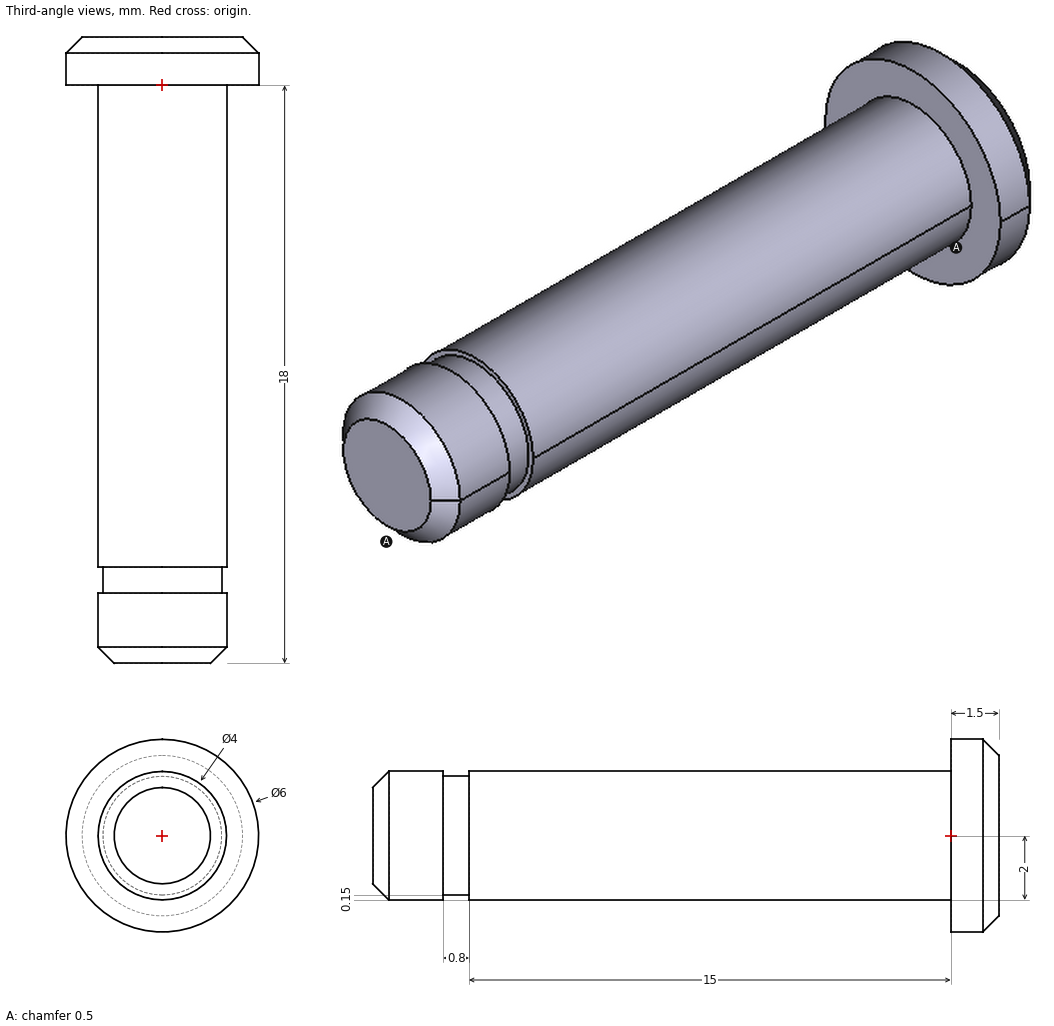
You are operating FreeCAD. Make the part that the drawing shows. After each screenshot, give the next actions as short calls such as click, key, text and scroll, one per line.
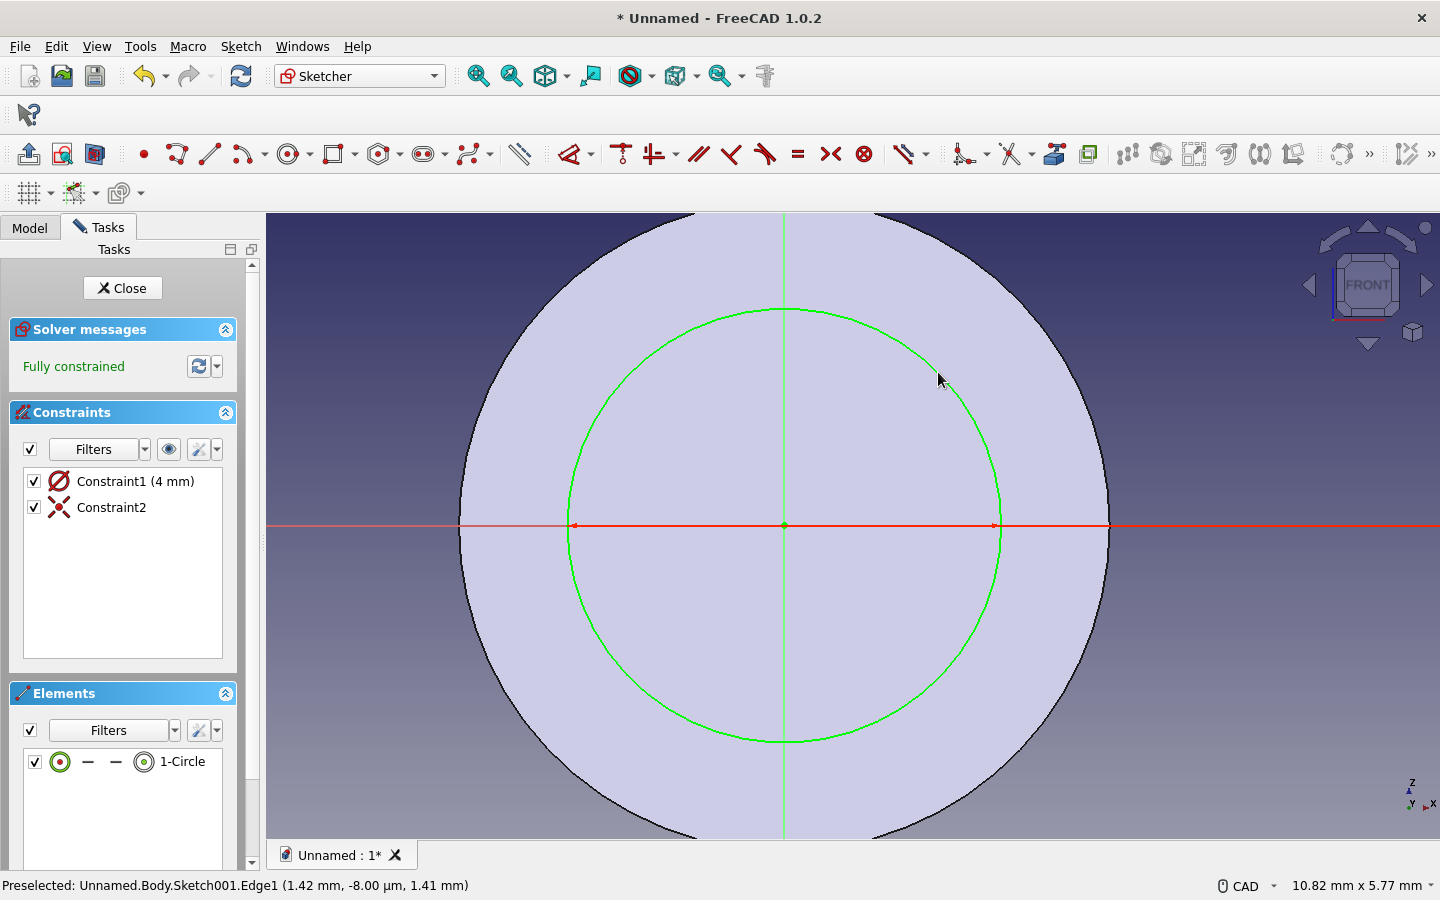
click(123, 288)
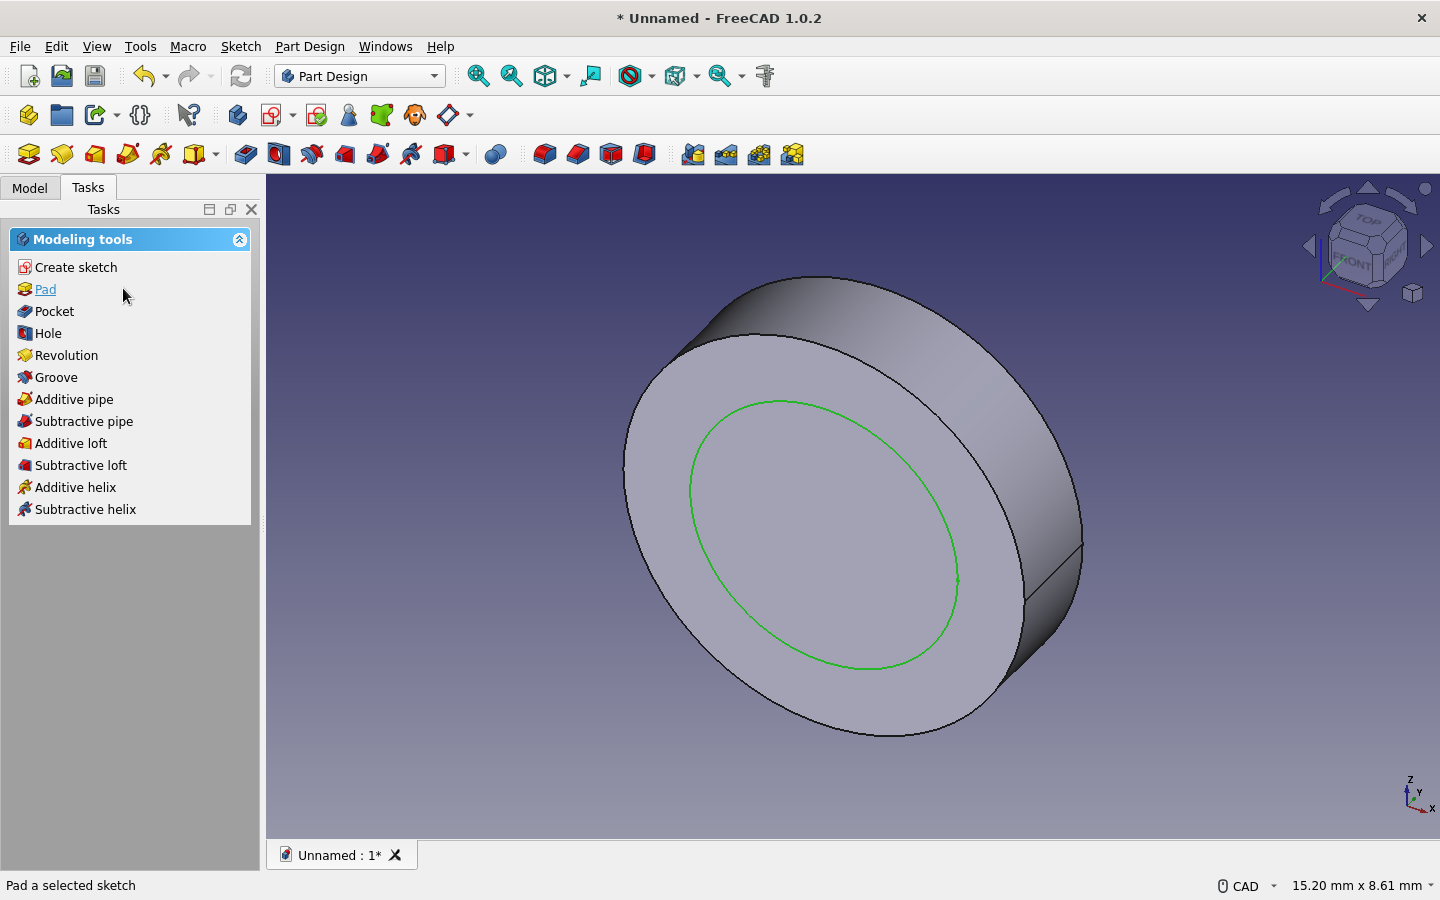
click(29, 154)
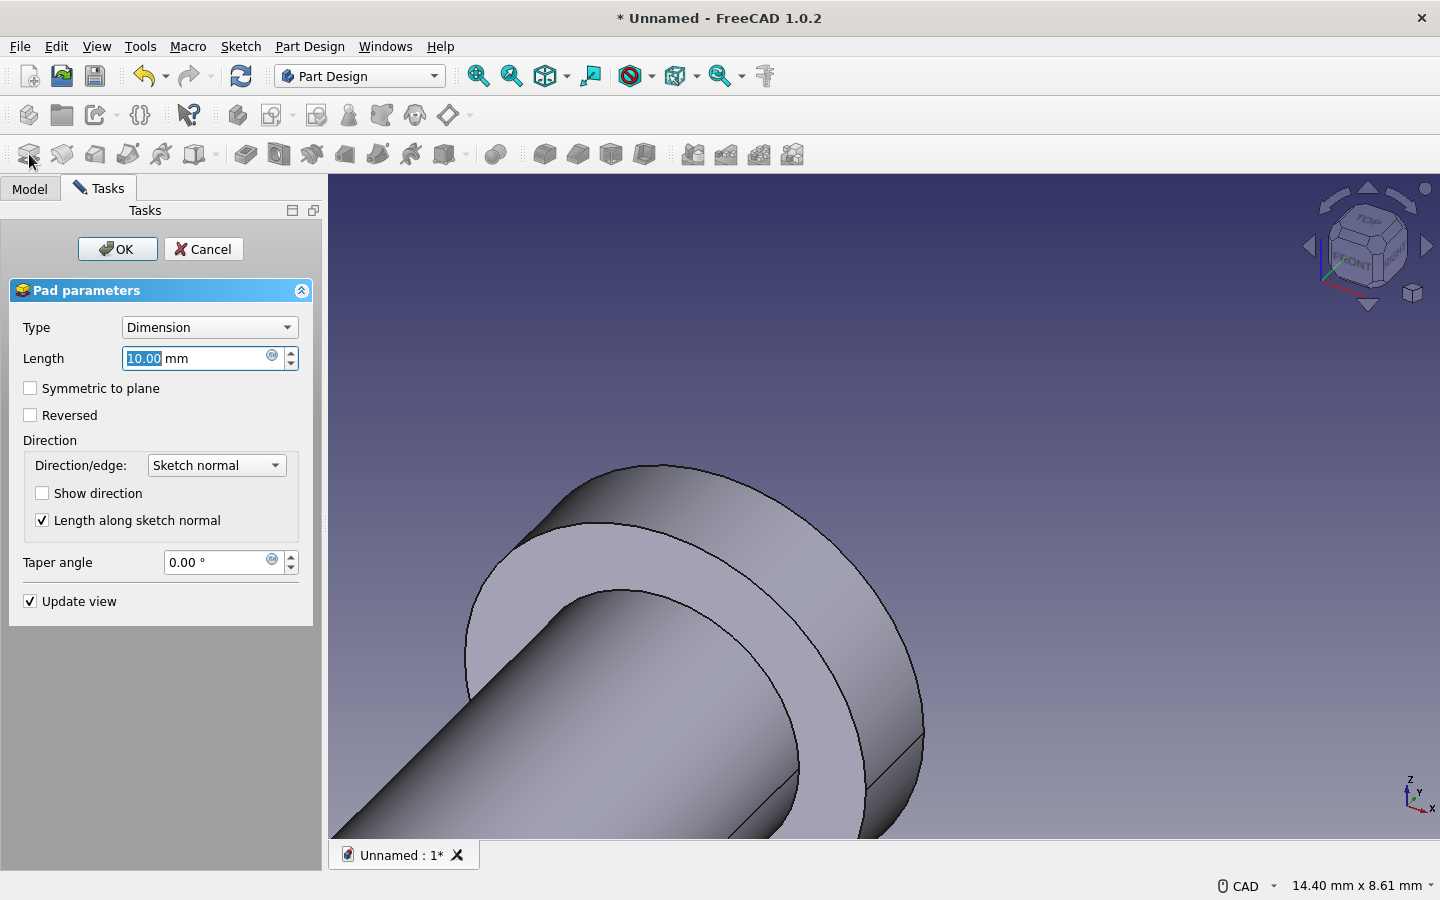
text(18)
key(Tab)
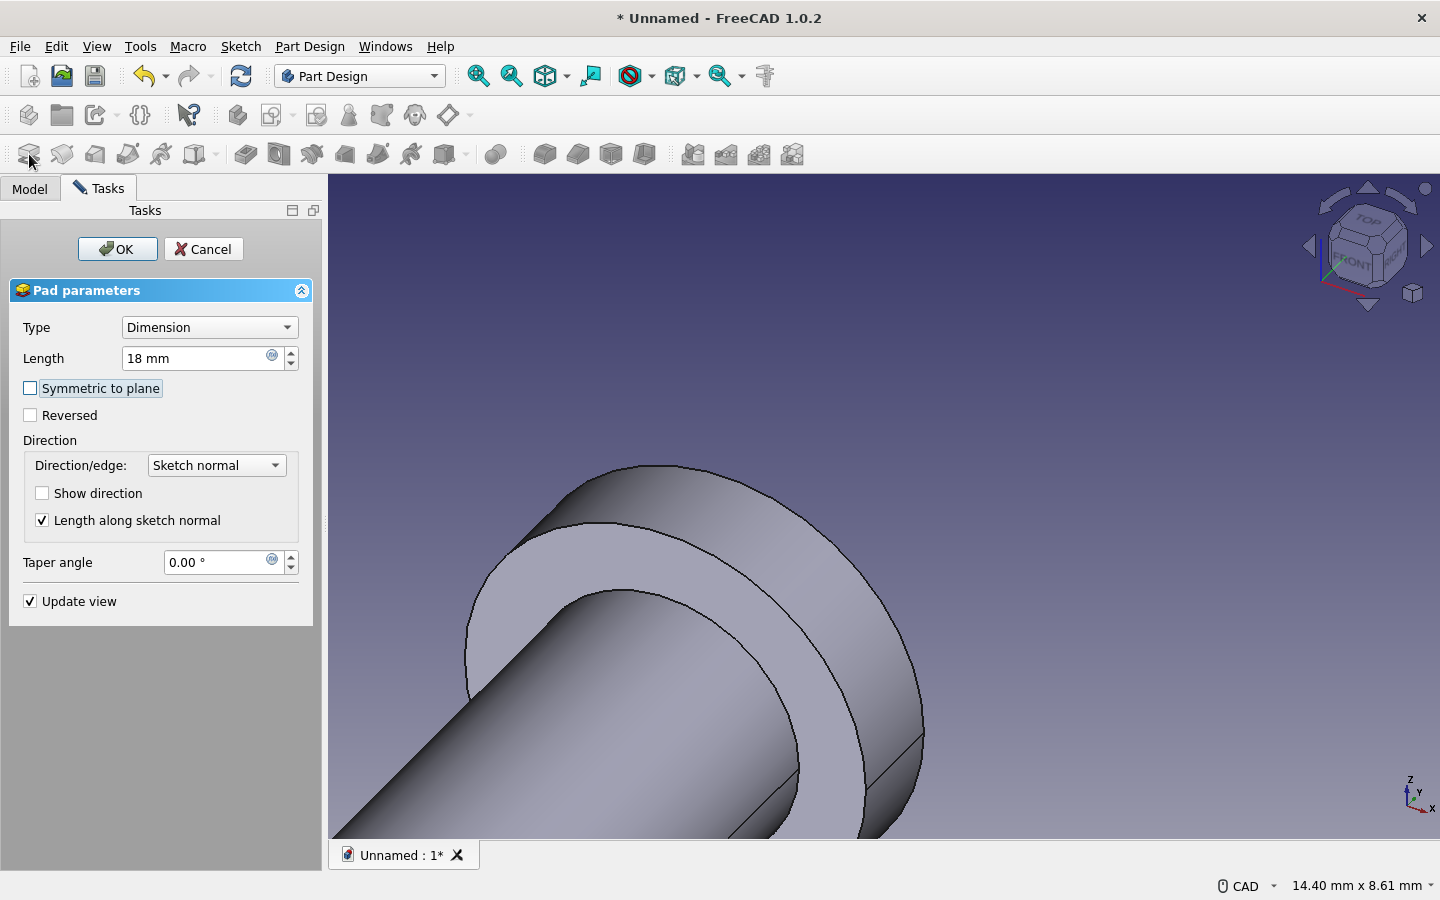
click(118, 249)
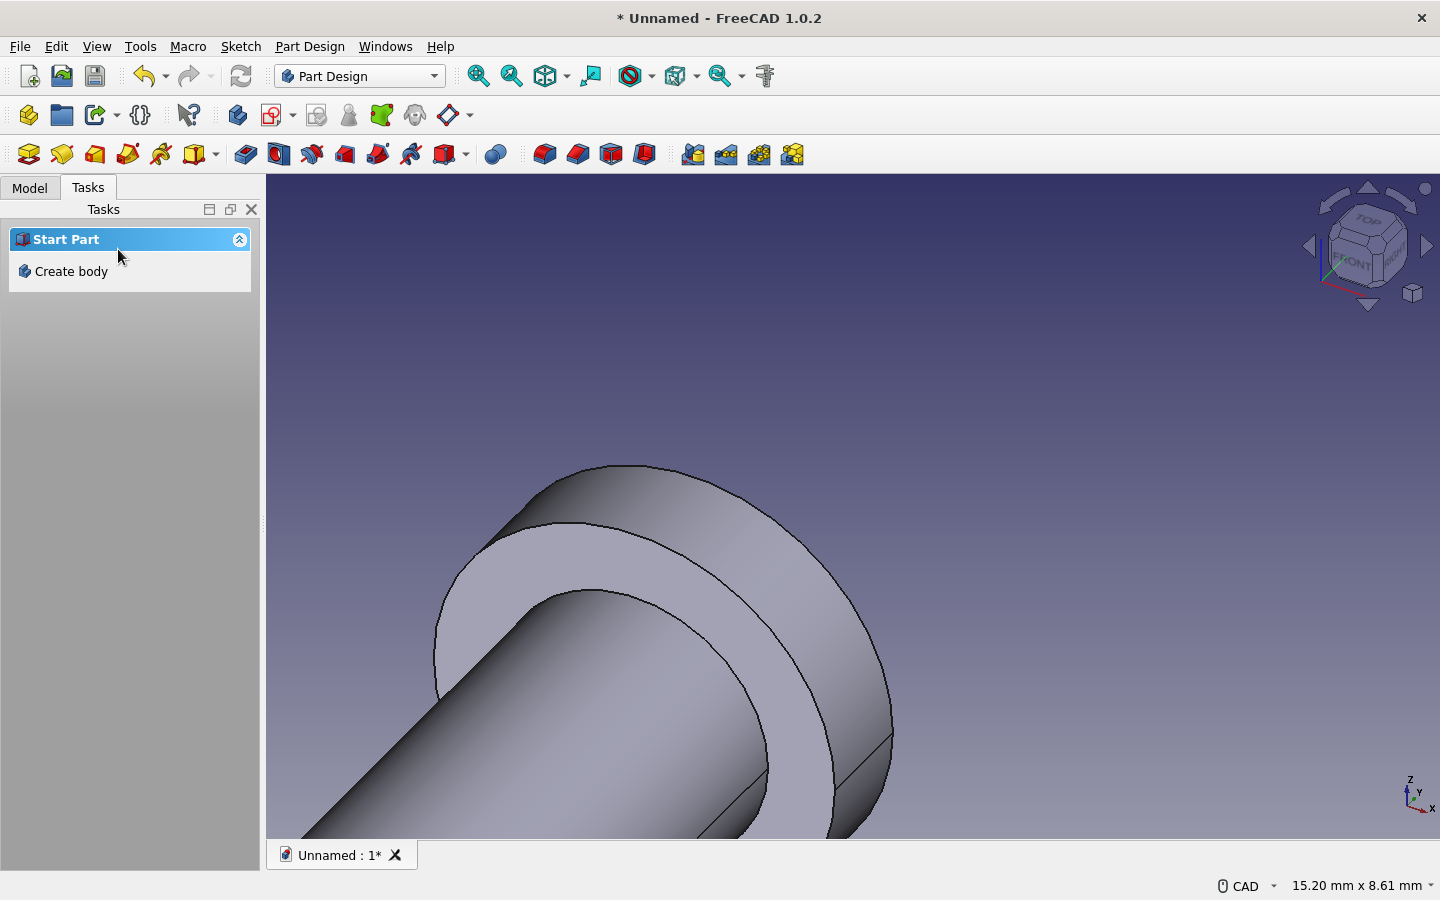
click(479, 76)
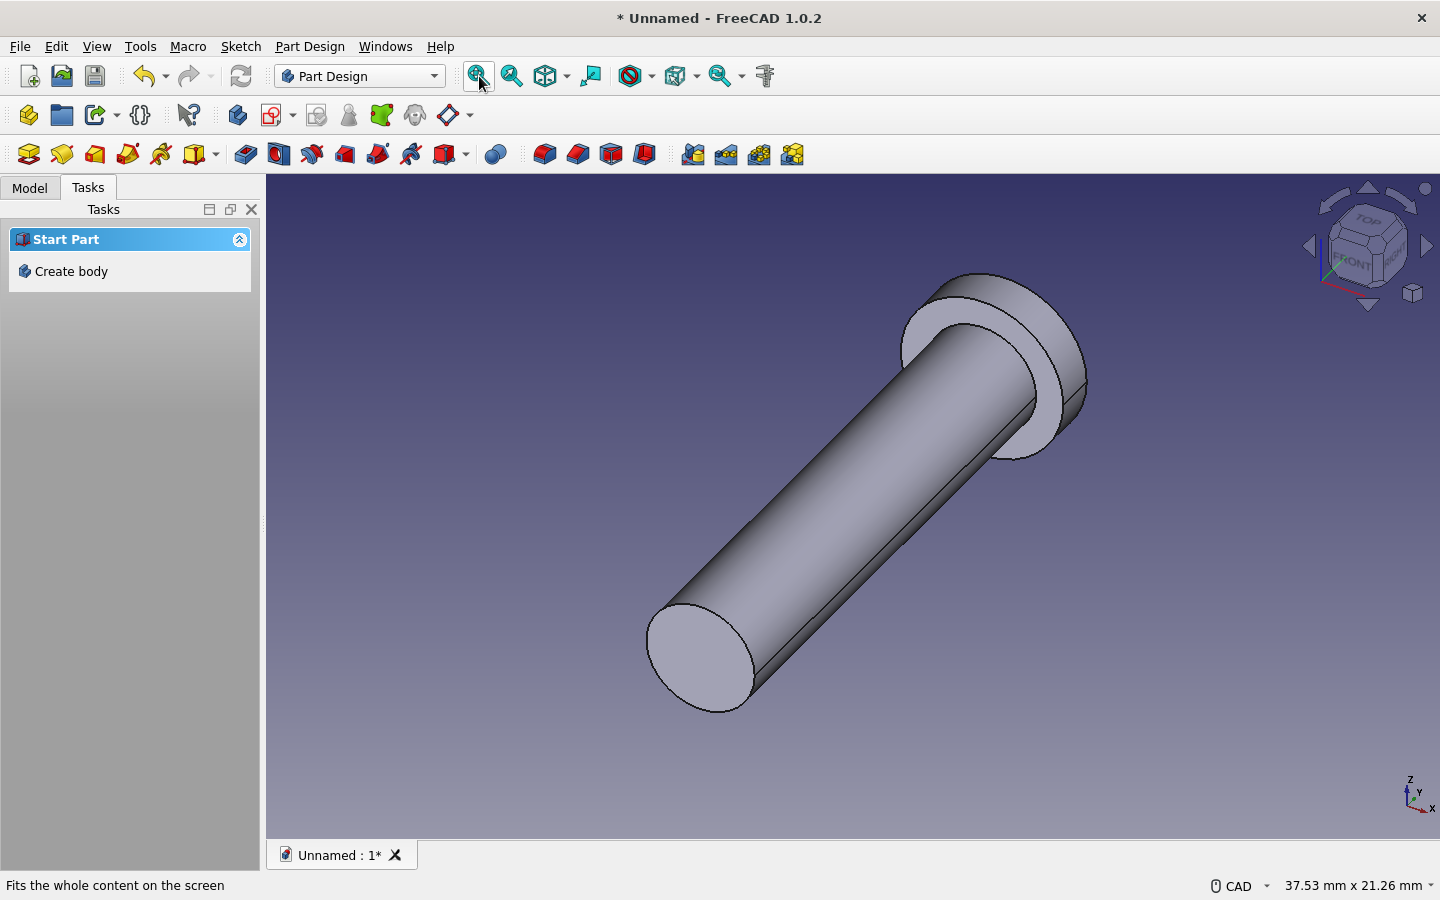
click(270, 116)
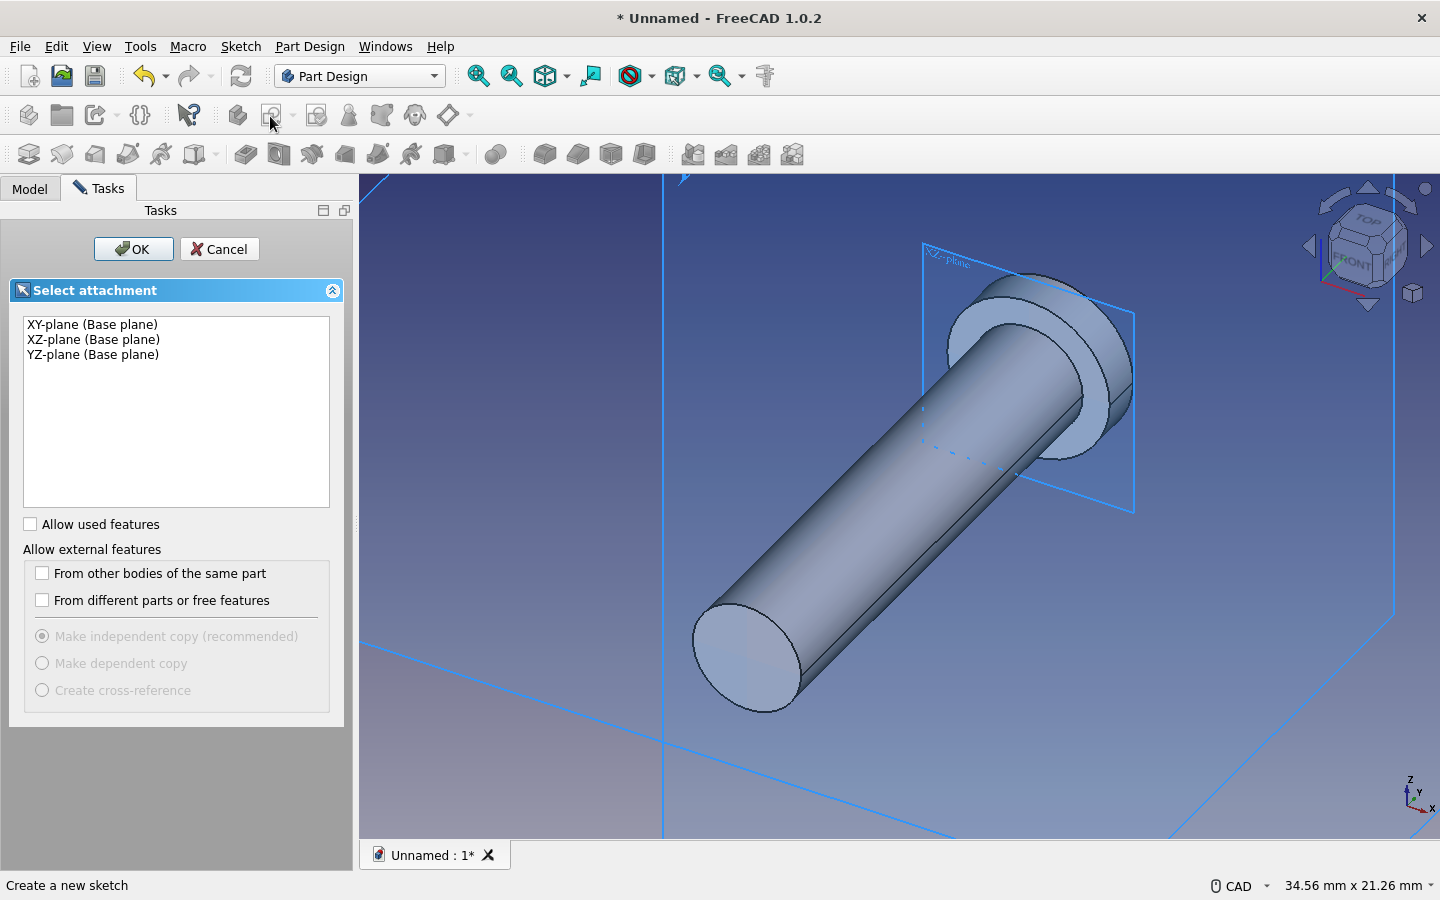
click(84, 354)